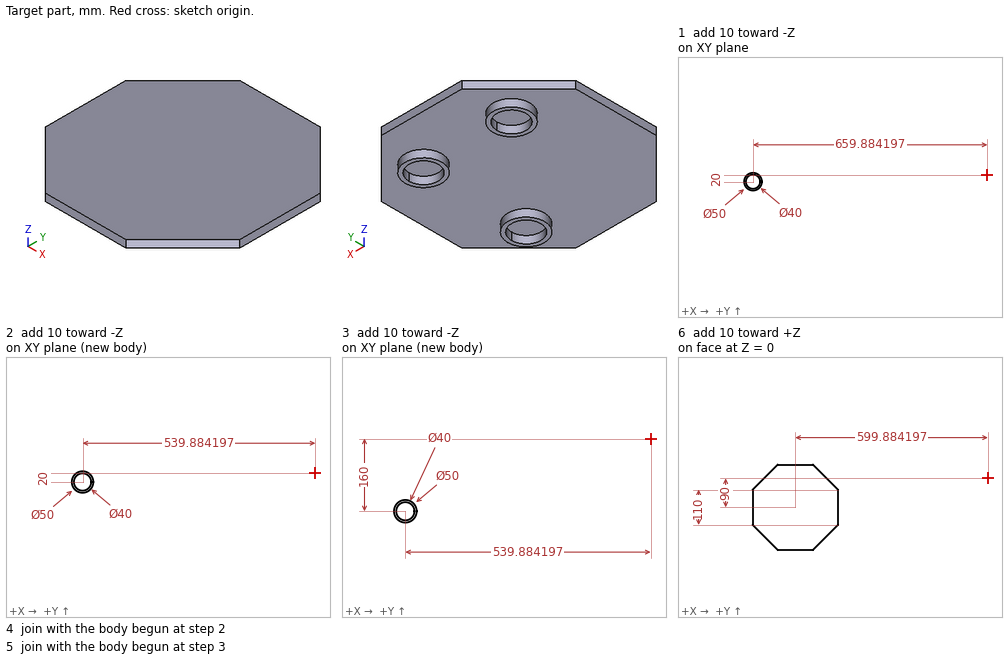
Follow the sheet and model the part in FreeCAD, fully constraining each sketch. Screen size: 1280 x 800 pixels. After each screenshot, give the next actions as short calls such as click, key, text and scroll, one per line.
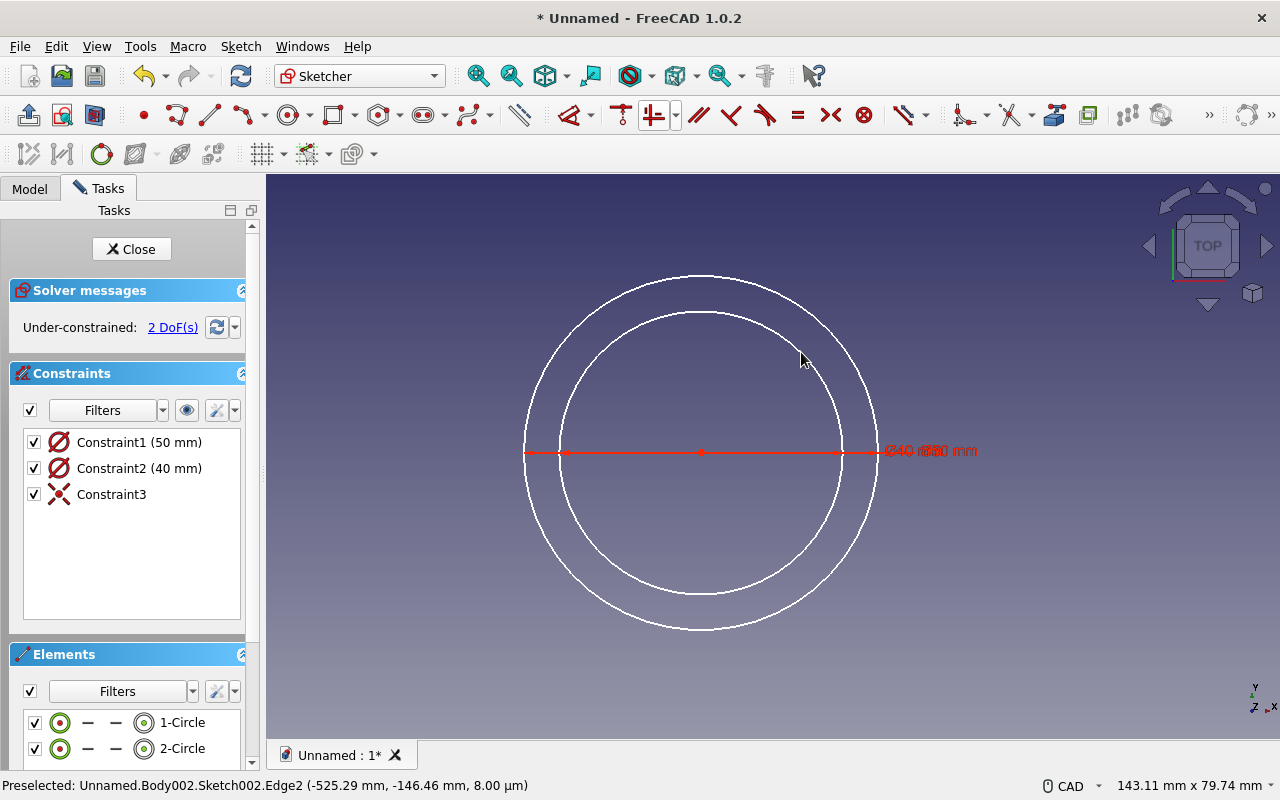
key(d)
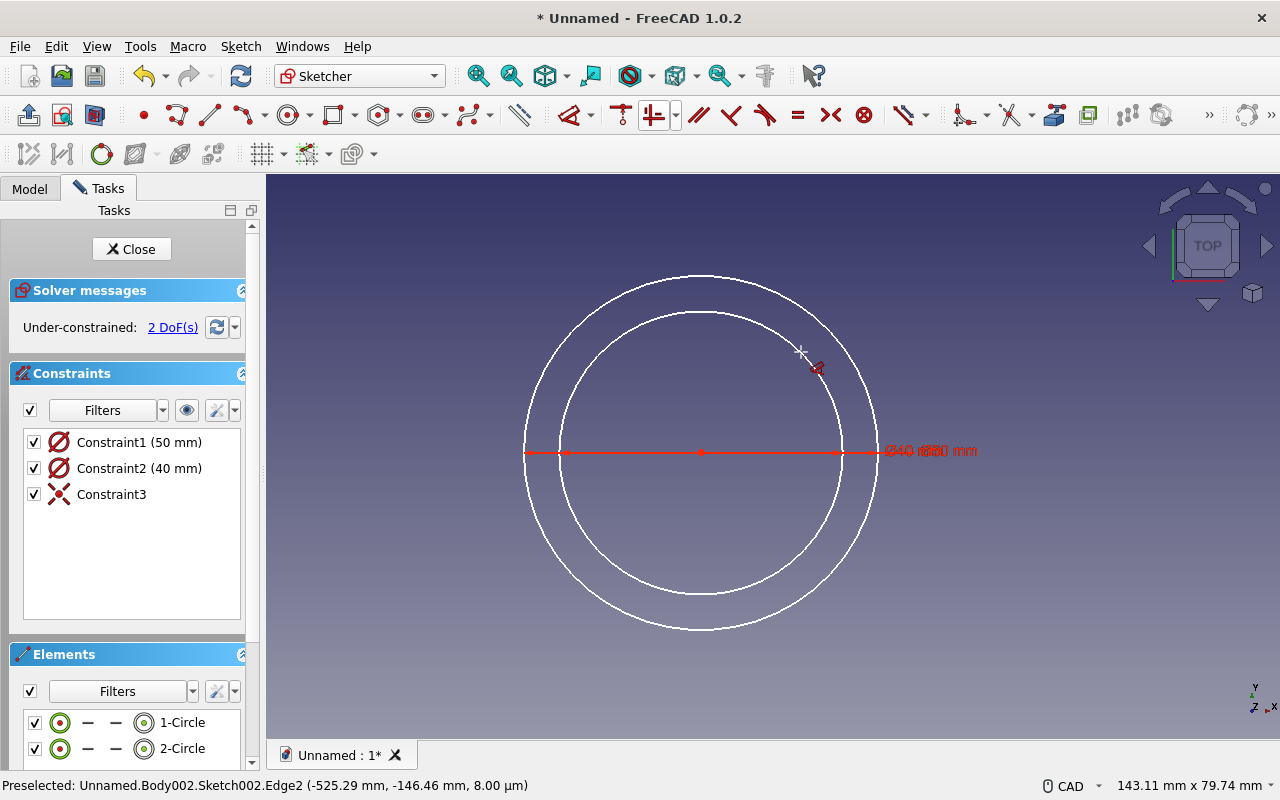
click(701, 453)
click(667, 385)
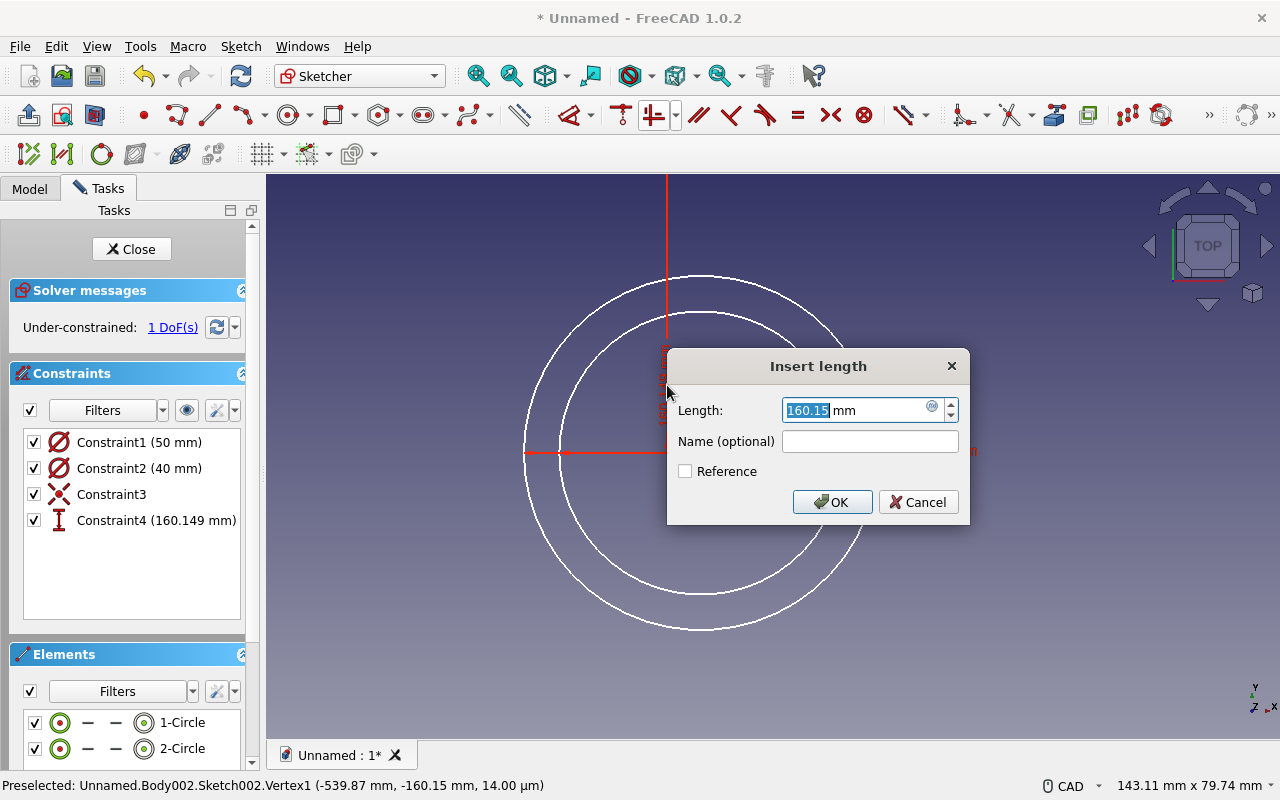
text(160)
key(Return)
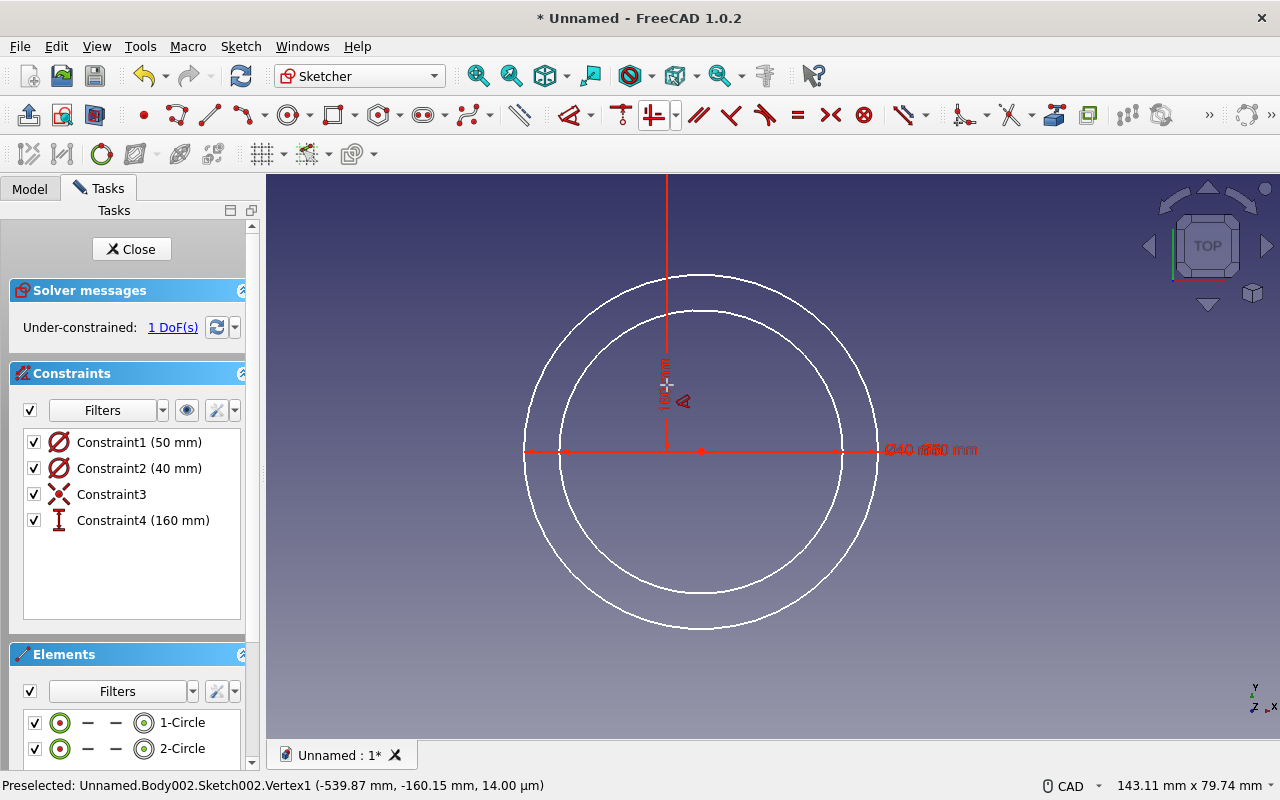
click(701, 452)
click(908, 486)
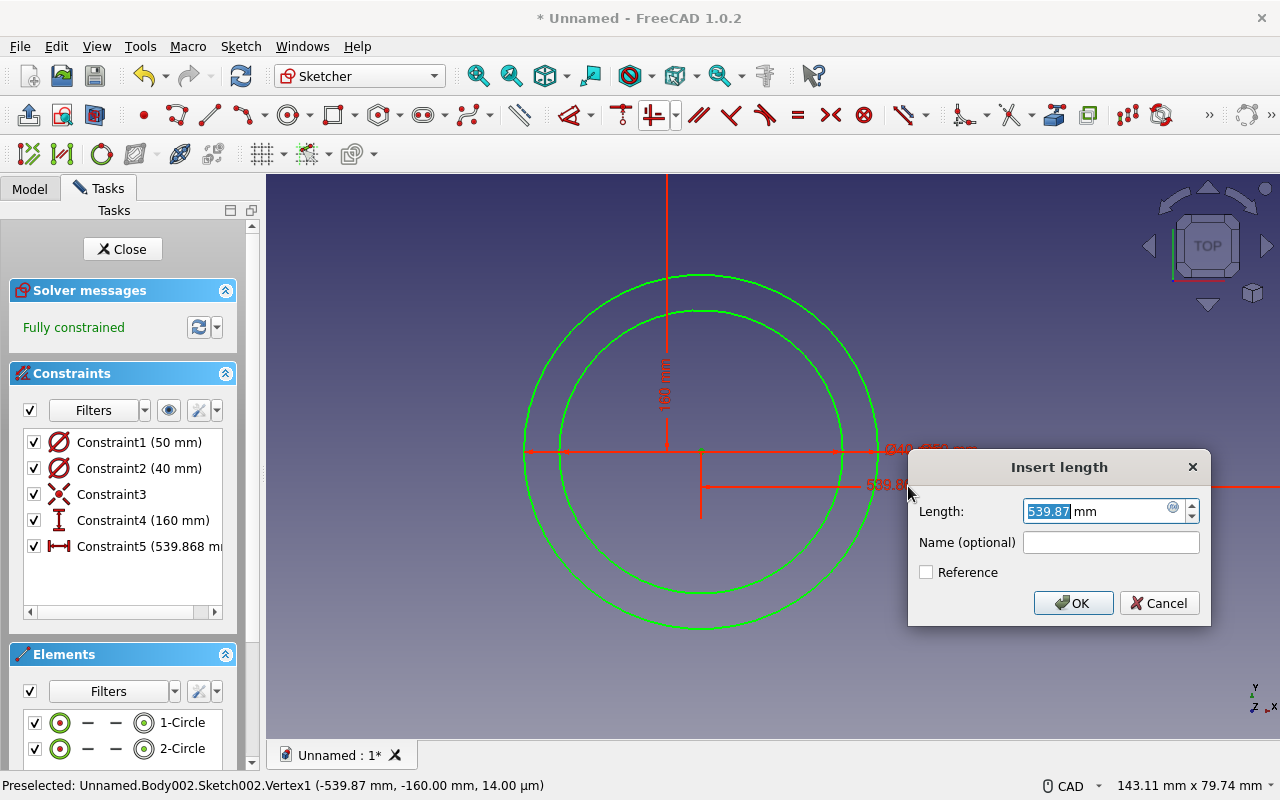
text(539.884197)
key(Return)
key(Escape)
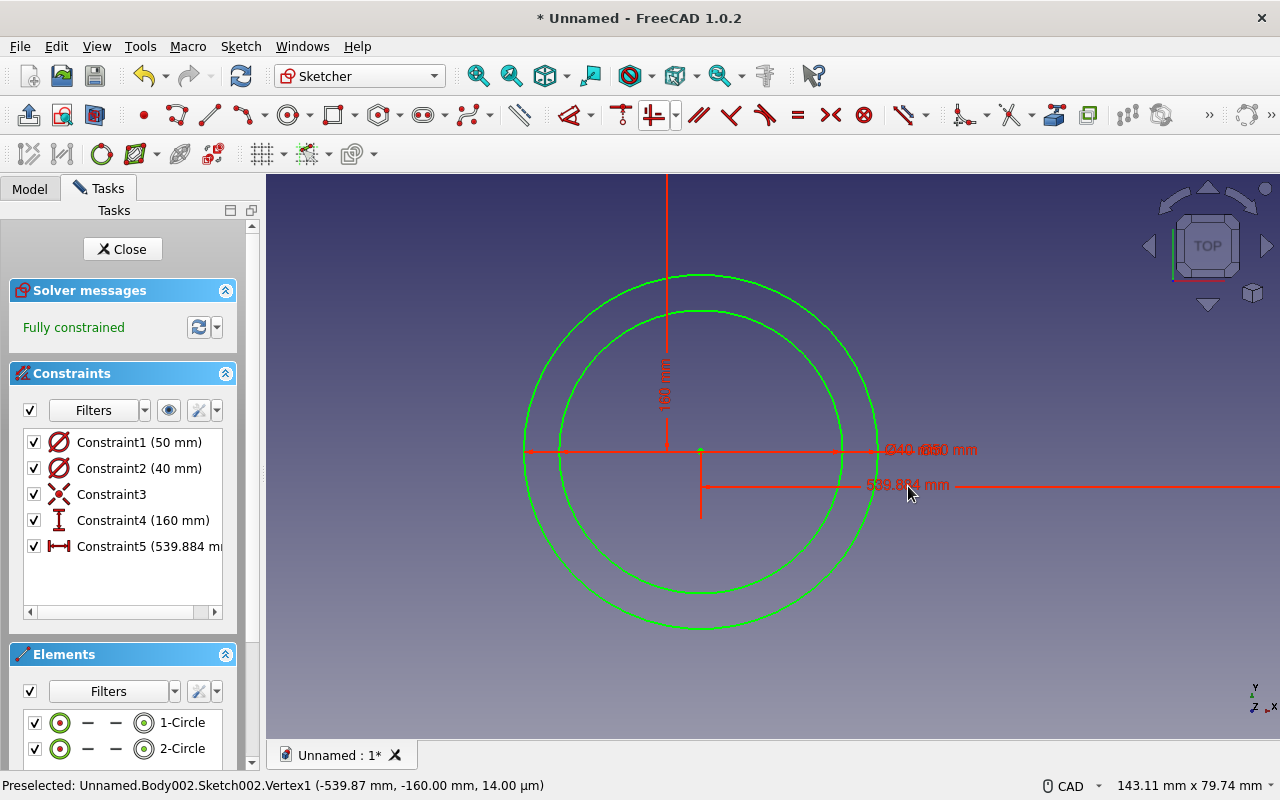
click(123, 249)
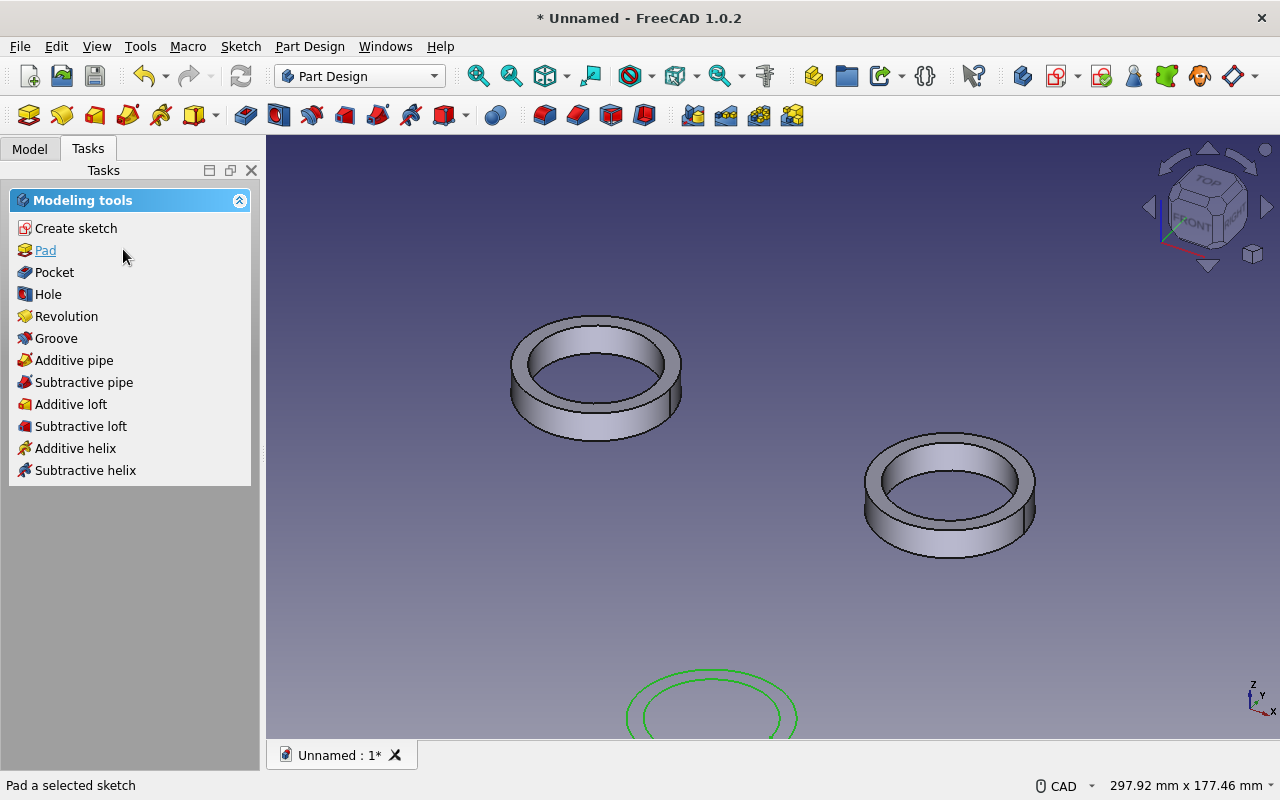
click(29, 116)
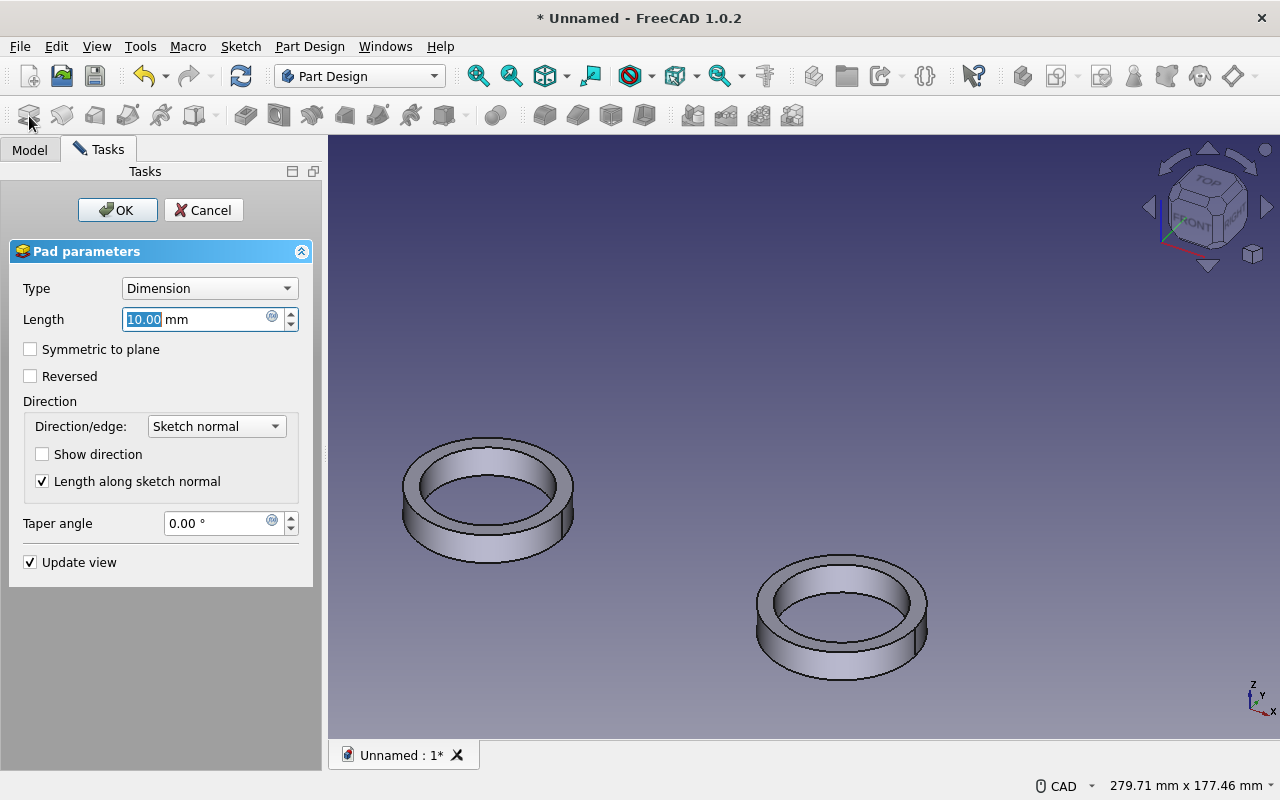
text(10)
key(Tab)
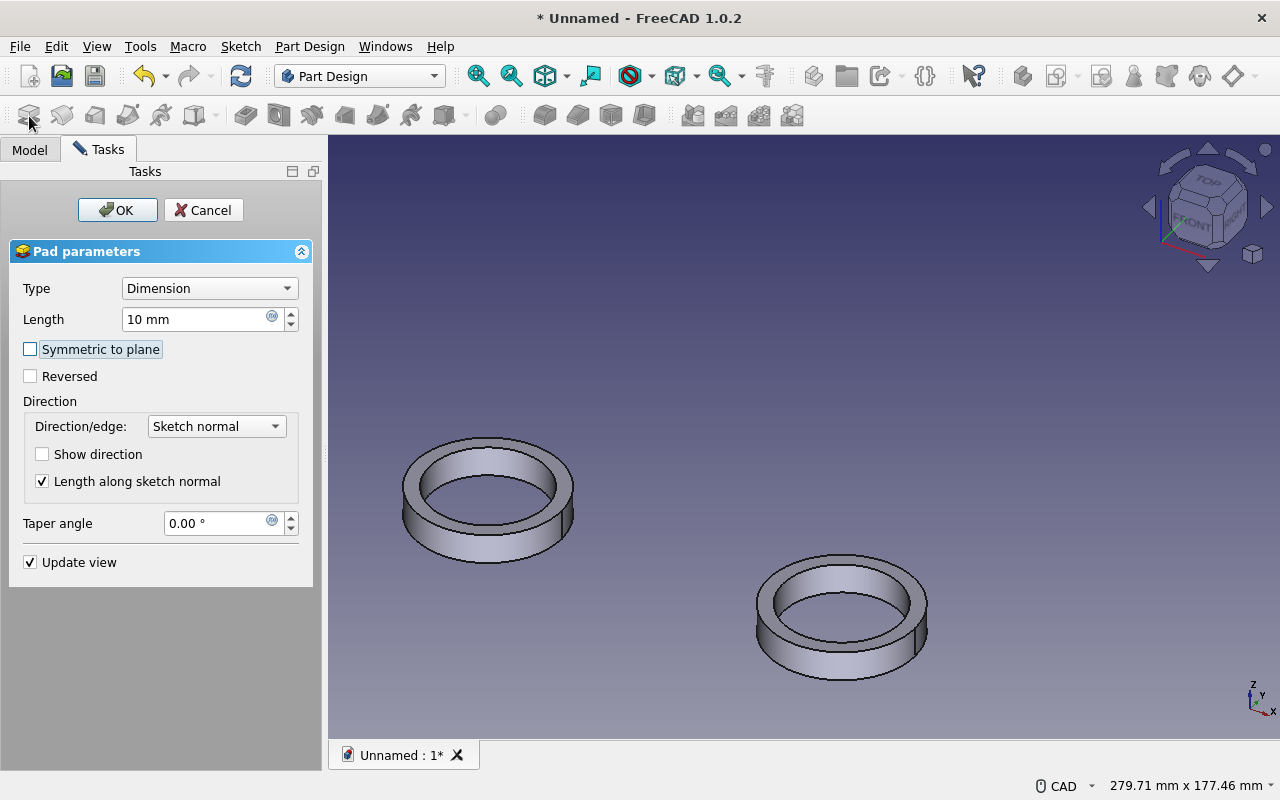
click(31, 376)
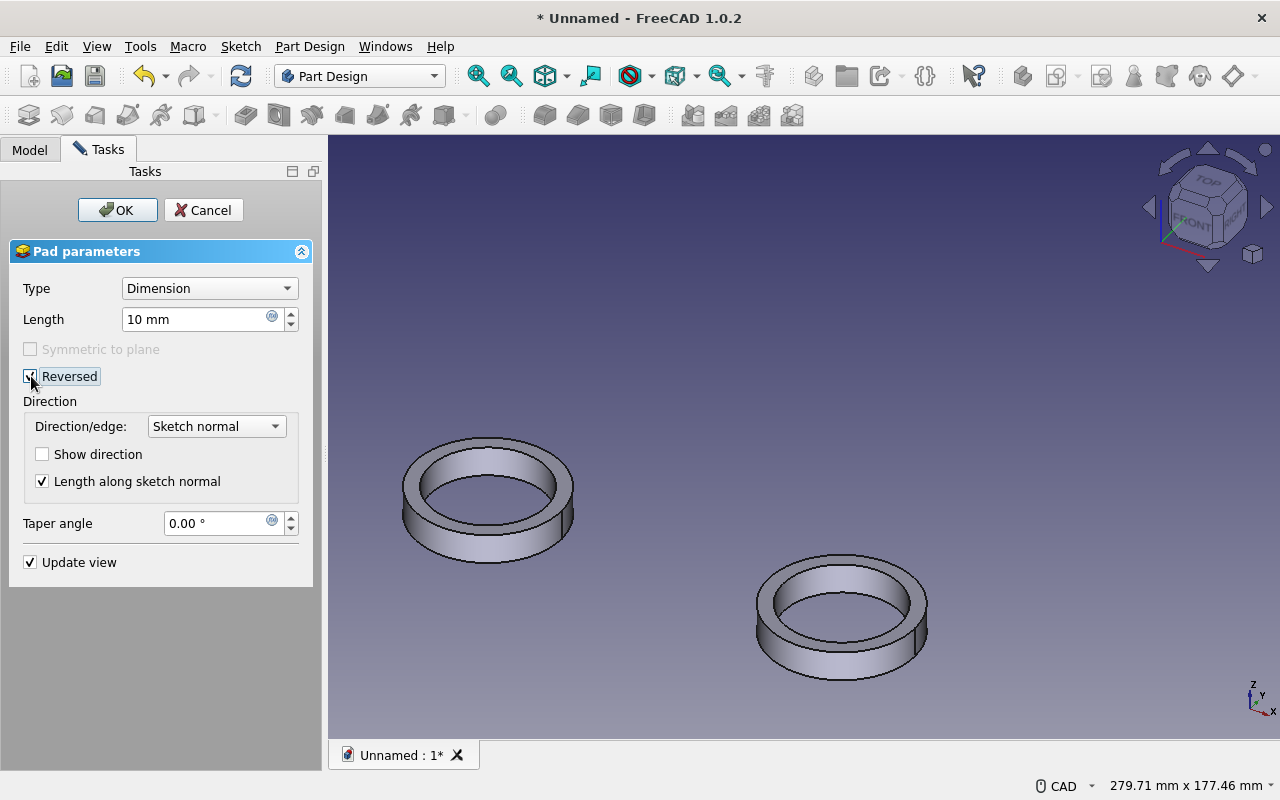
click(118, 210)